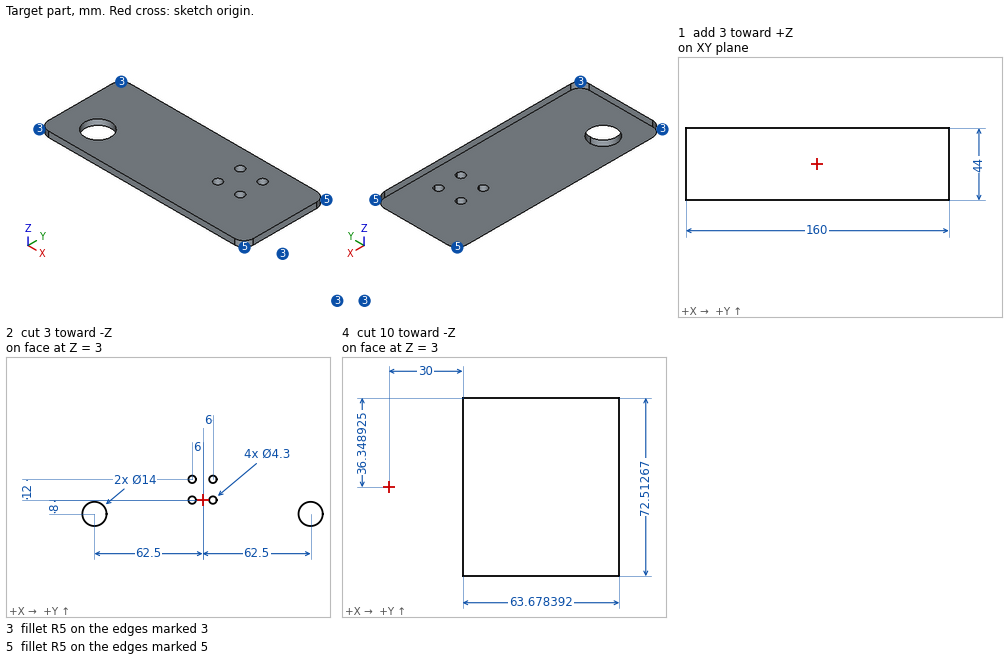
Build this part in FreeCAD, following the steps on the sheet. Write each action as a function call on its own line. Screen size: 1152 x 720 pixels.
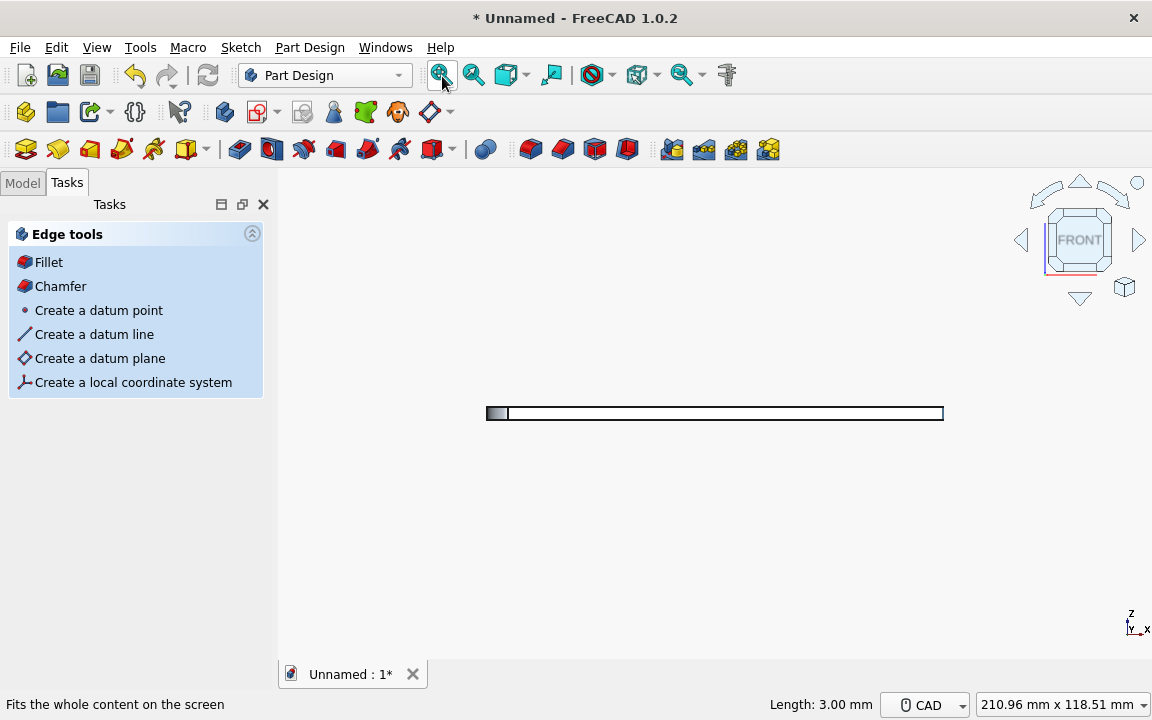
key(3)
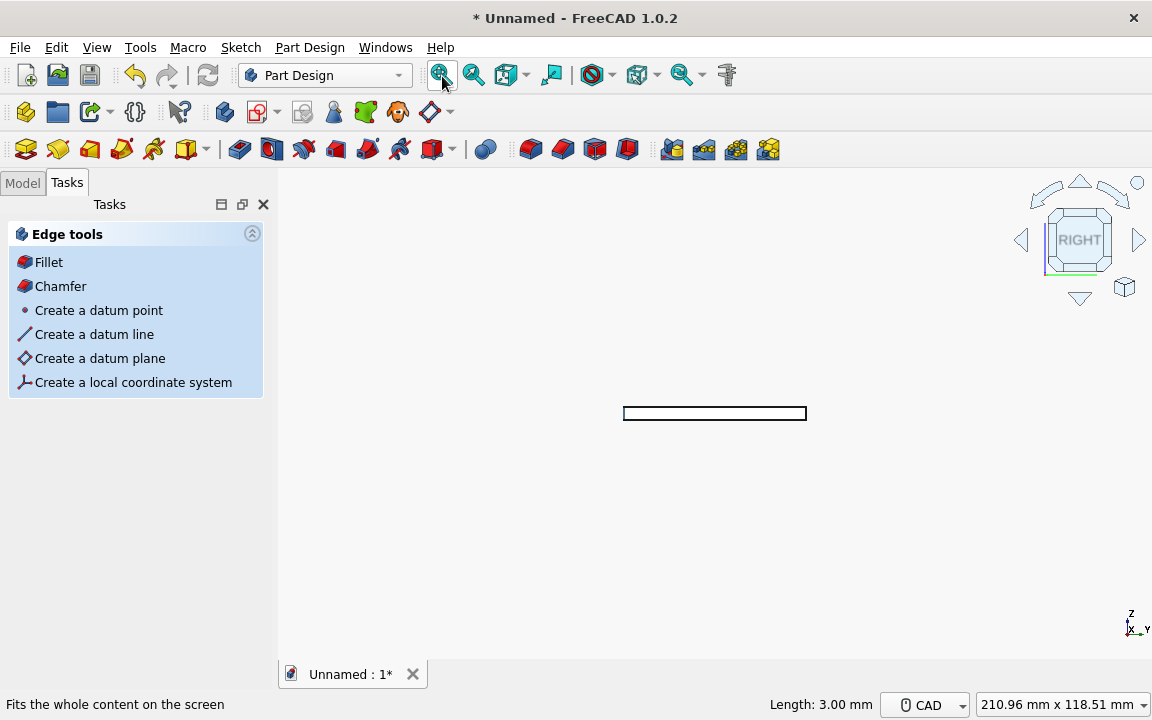
click(442, 76)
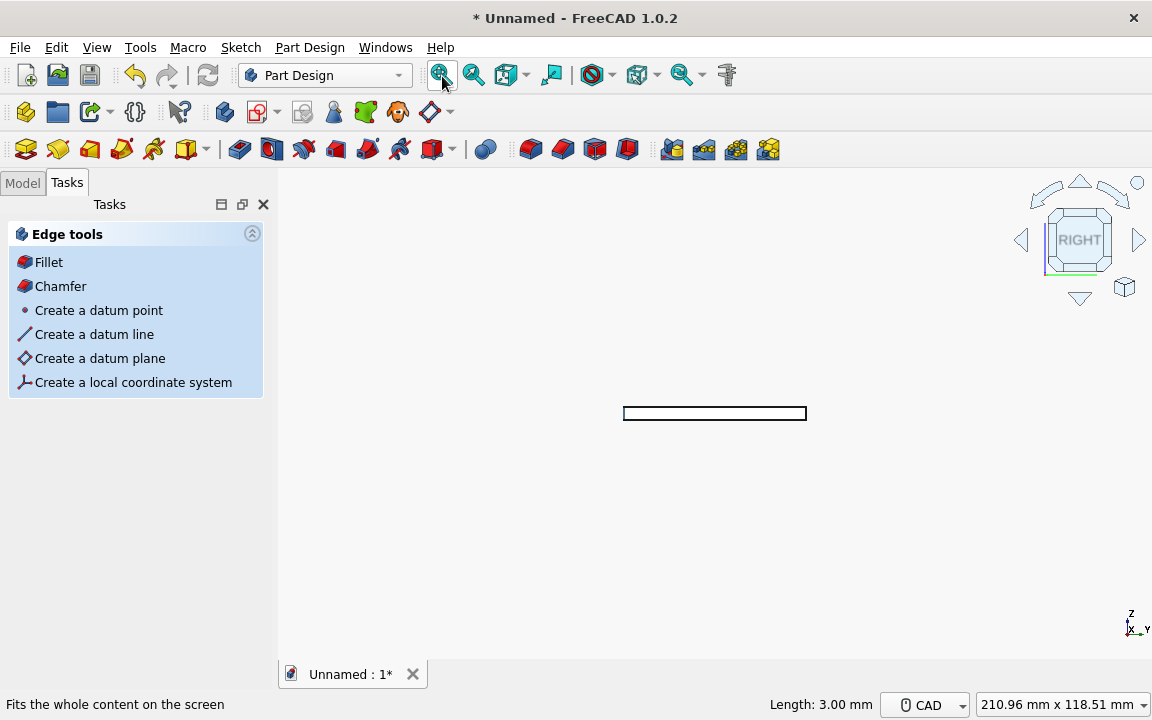
scroll(806, 412, up, 6)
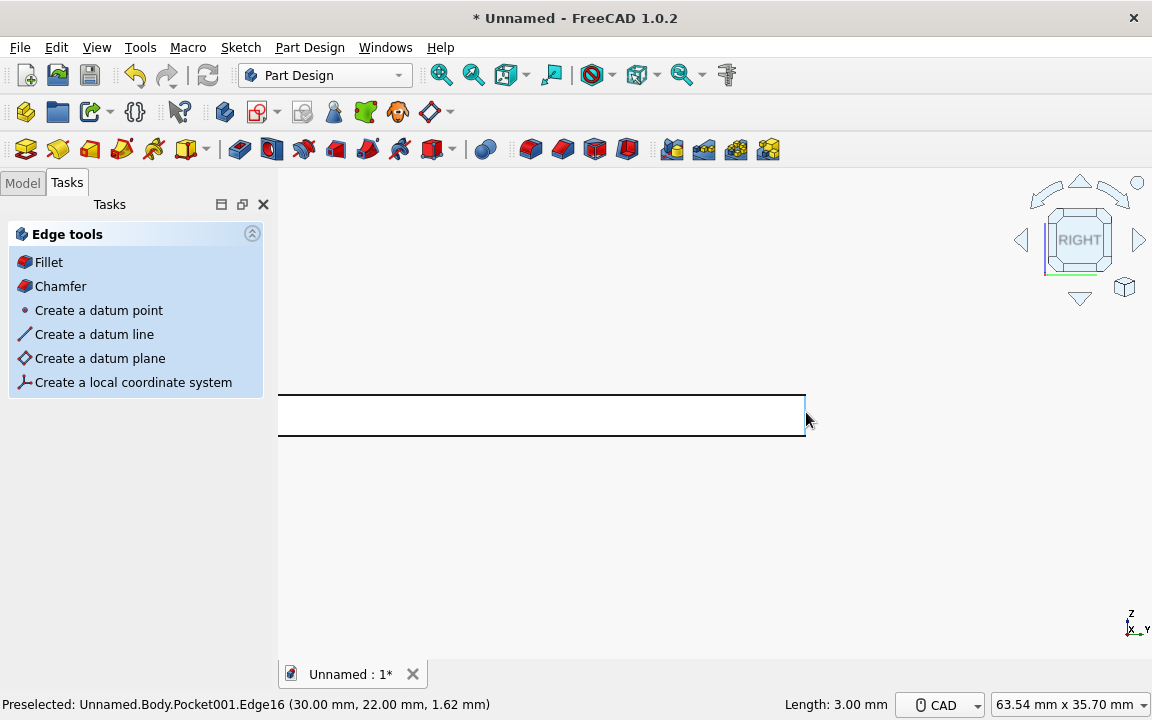
click(805, 415, ctrl)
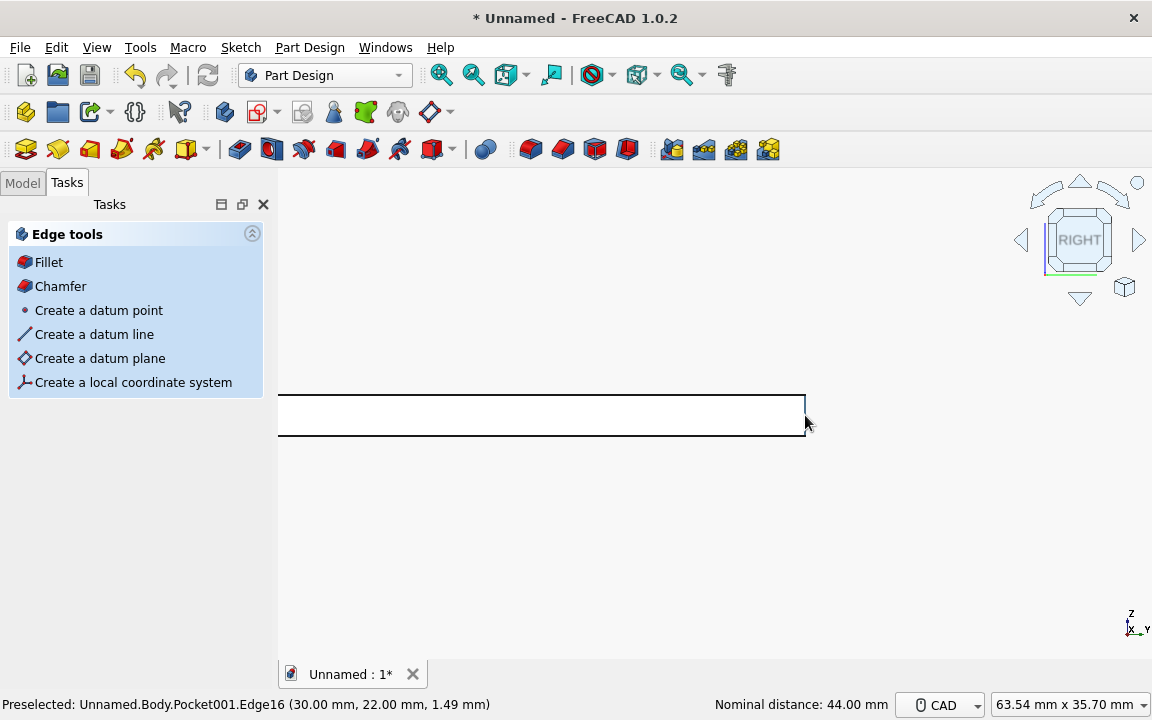
click(532, 150)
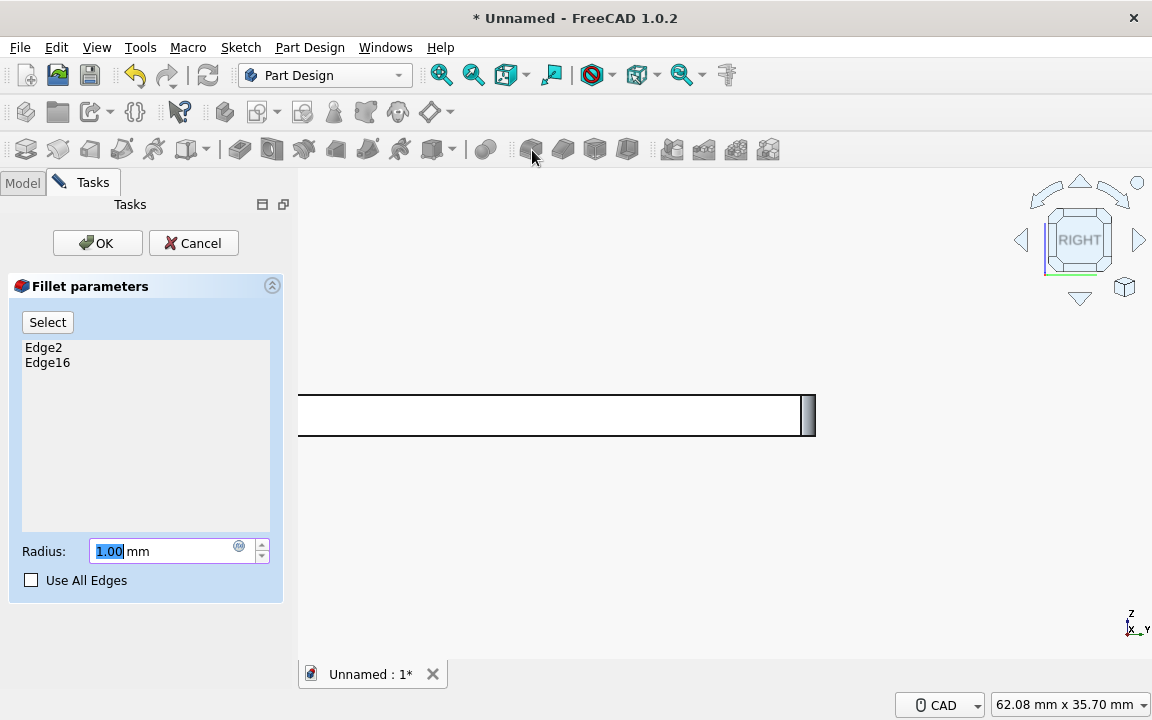
text(5)
key(Tab)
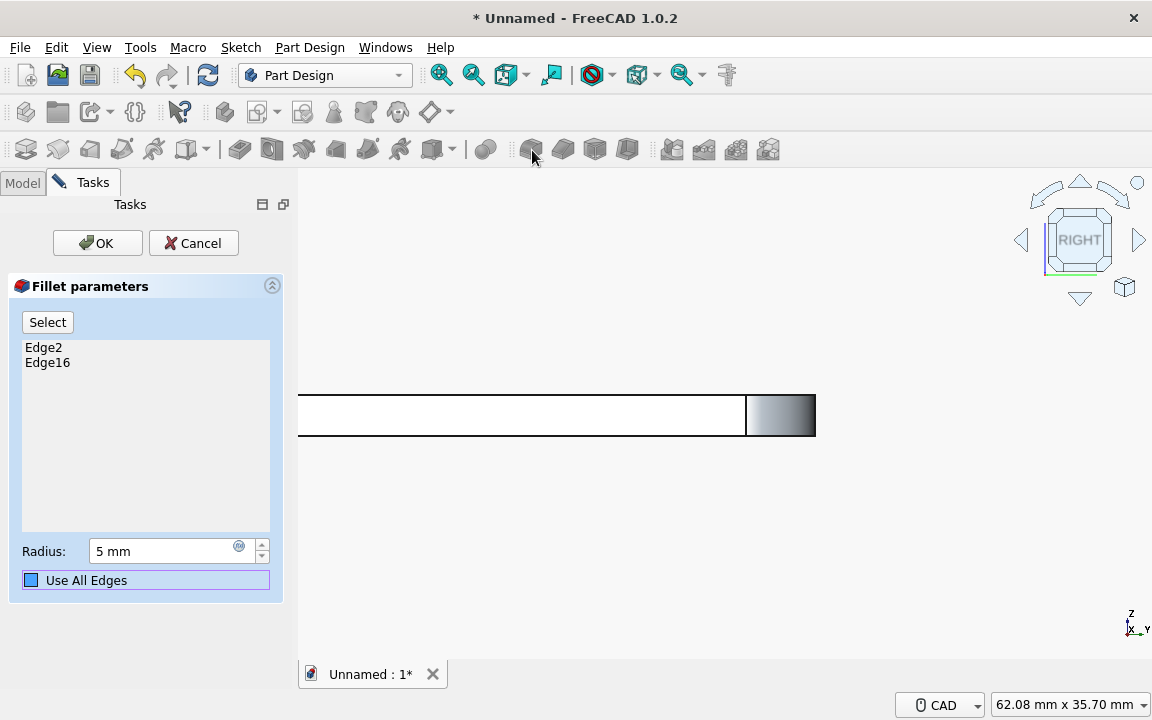
click(98, 243)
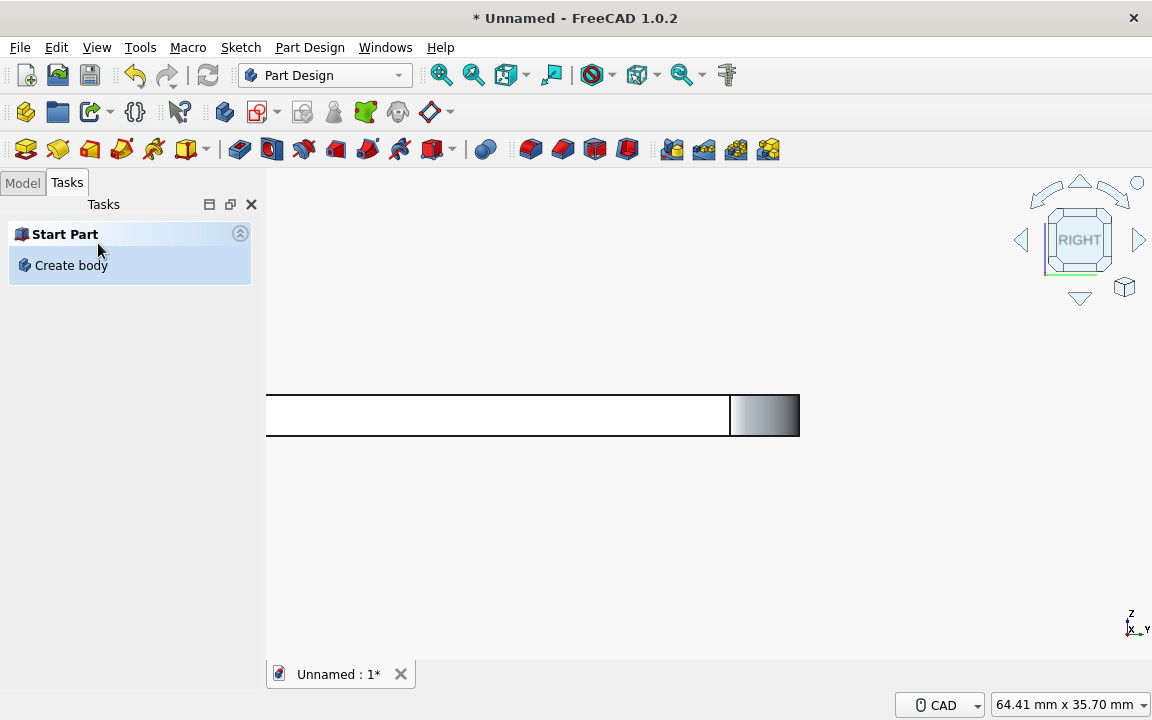
key(0)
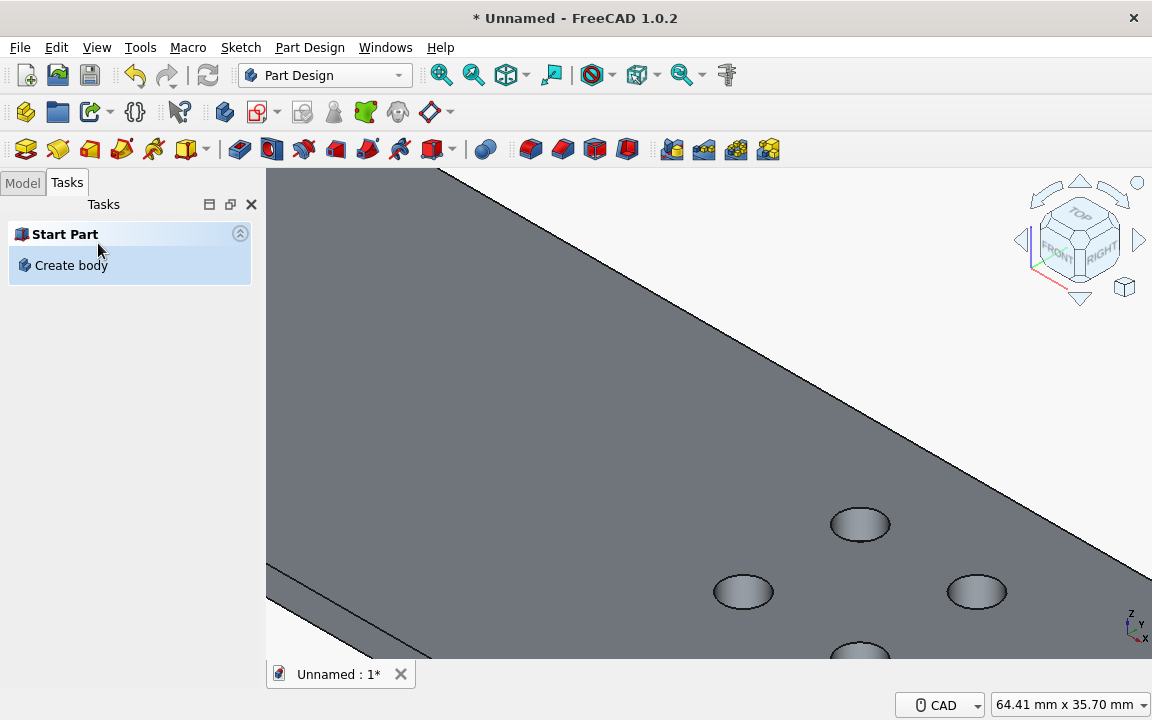
key(v)
key(f)